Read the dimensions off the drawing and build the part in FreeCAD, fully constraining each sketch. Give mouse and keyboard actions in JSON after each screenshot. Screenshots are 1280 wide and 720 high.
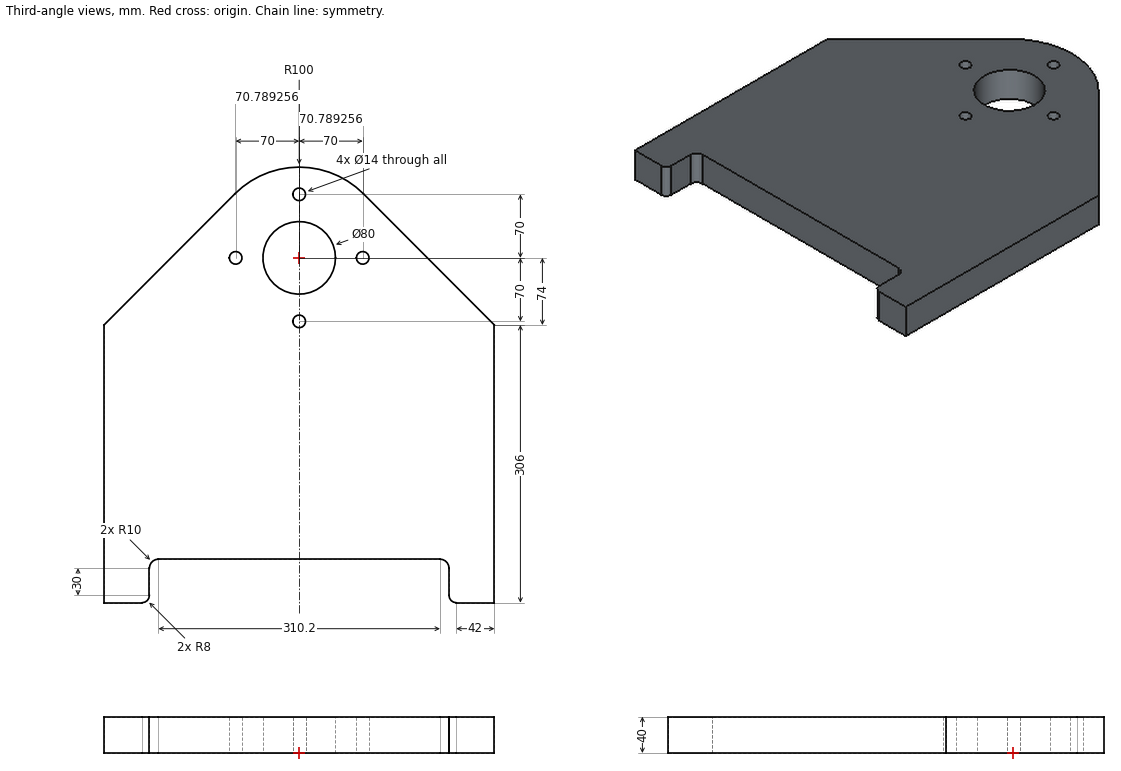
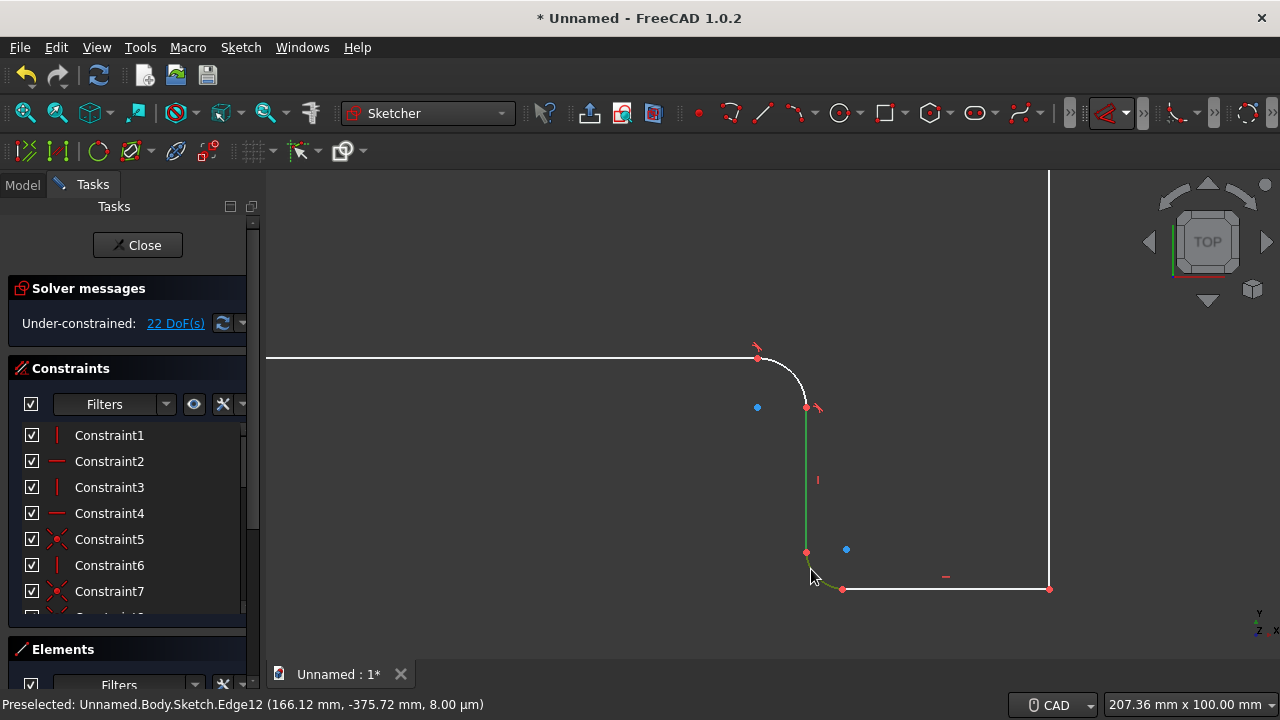
{"action": "key", "text": "t"}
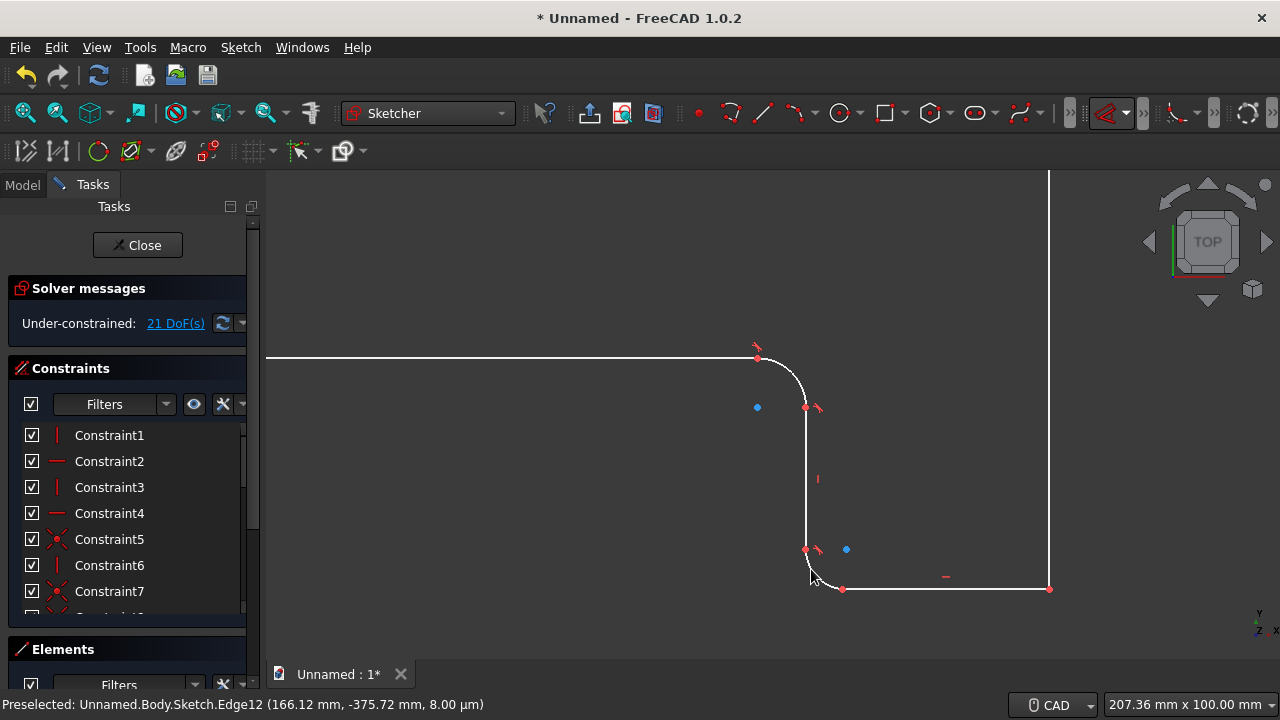
{"action": "scroll", "coordinate": [815, 571], "scroll_direction": "down", "scroll_amount": 10}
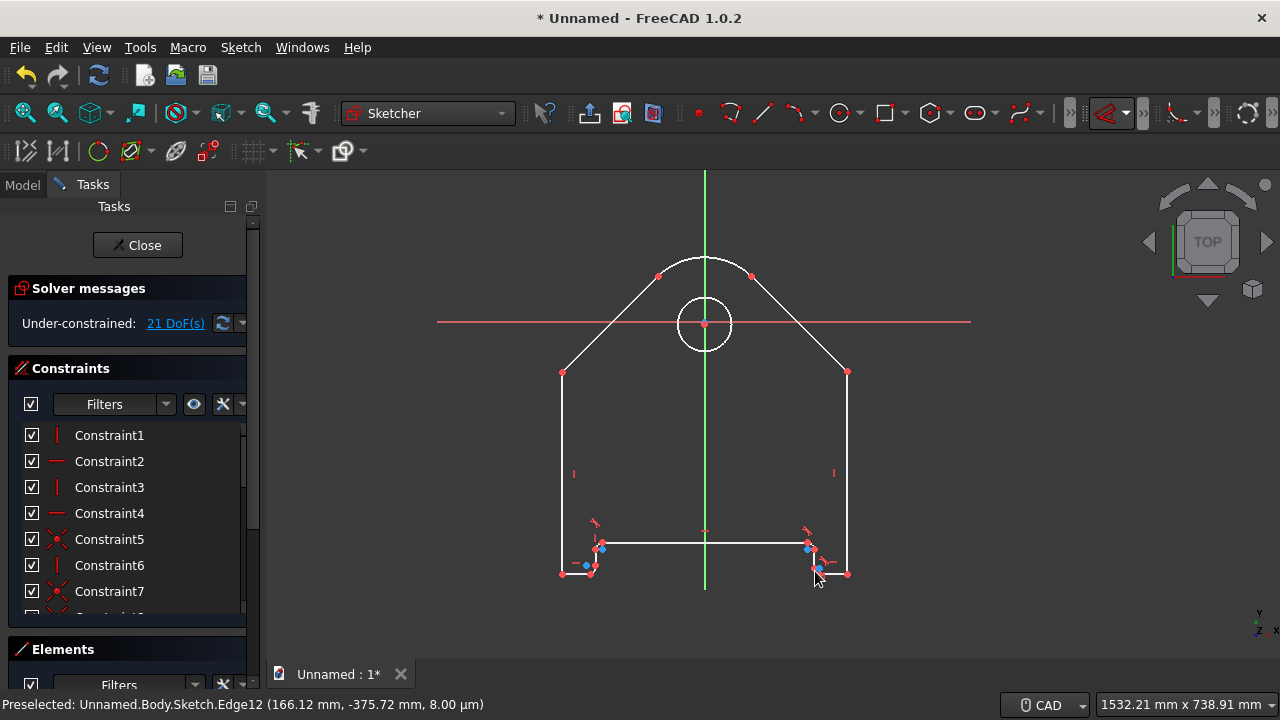
{"action": "scroll", "coordinate": [828, 574], "scroll_direction": "up", "scroll_amount": 3}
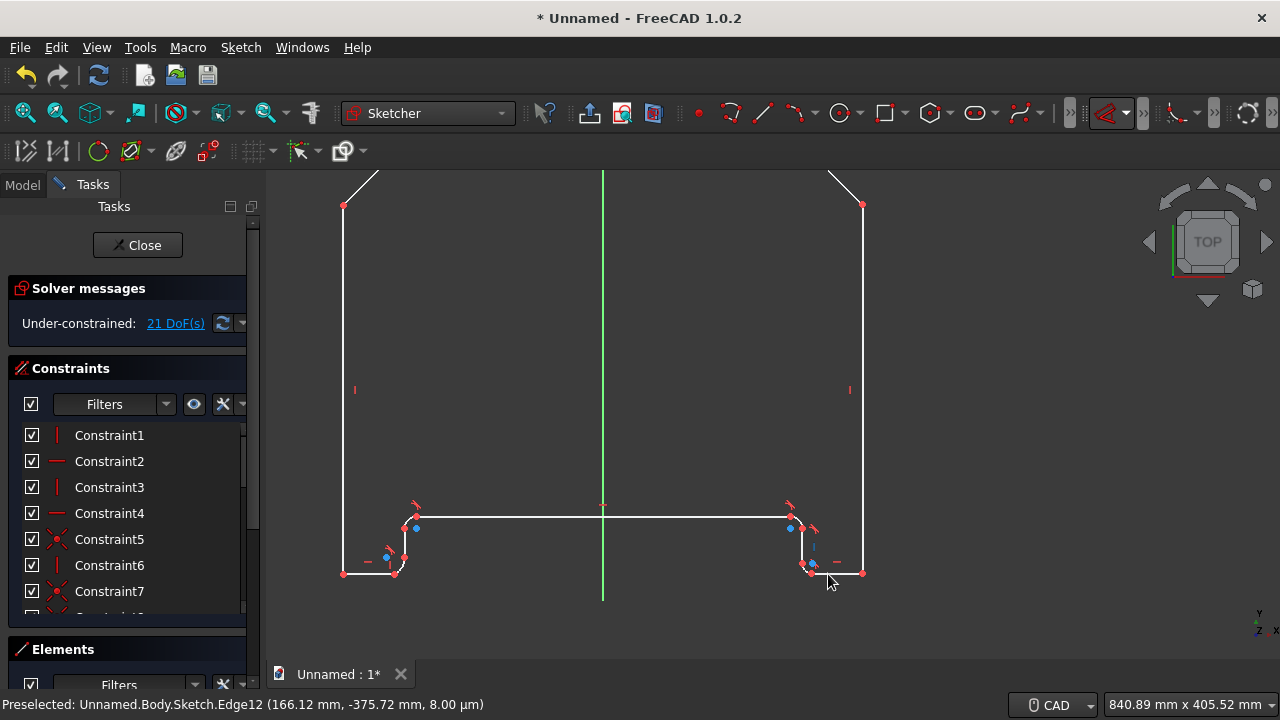
{"action": "left_click", "coordinate": [827, 574]}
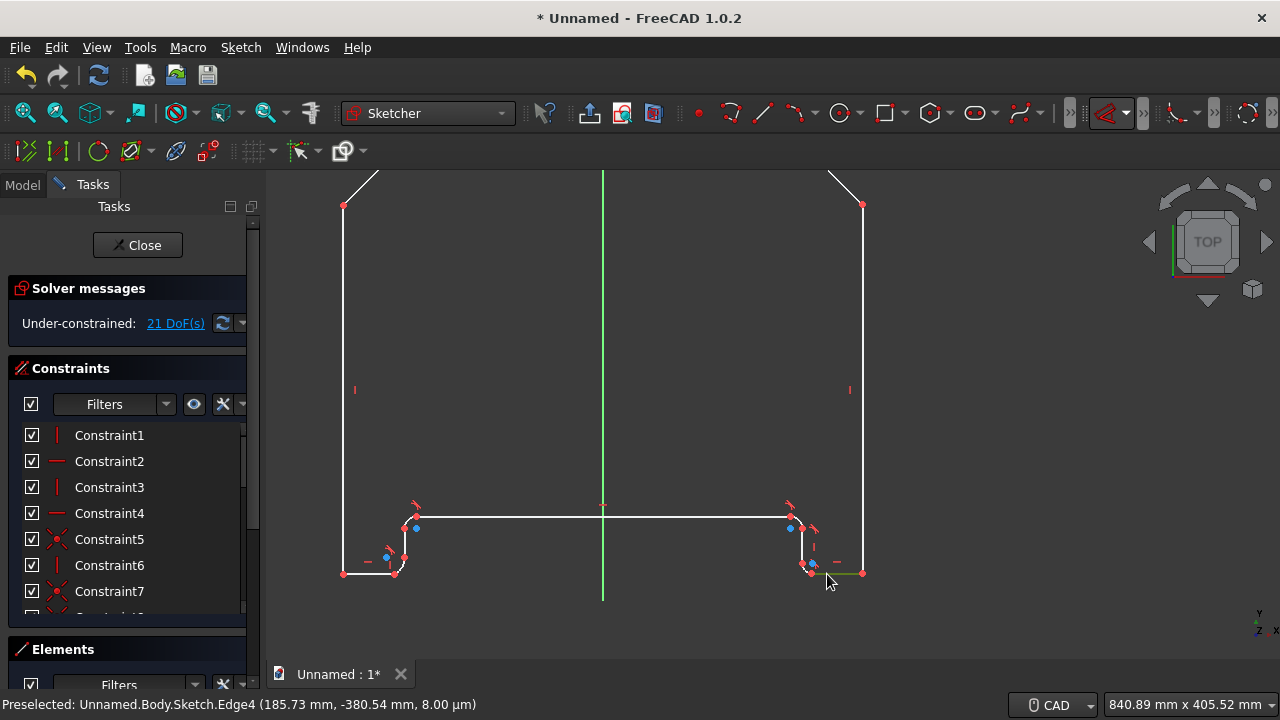
{"action": "scroll", "coordinate": [805, 570], "scroll_direction": "up", "scroll_amount": 4}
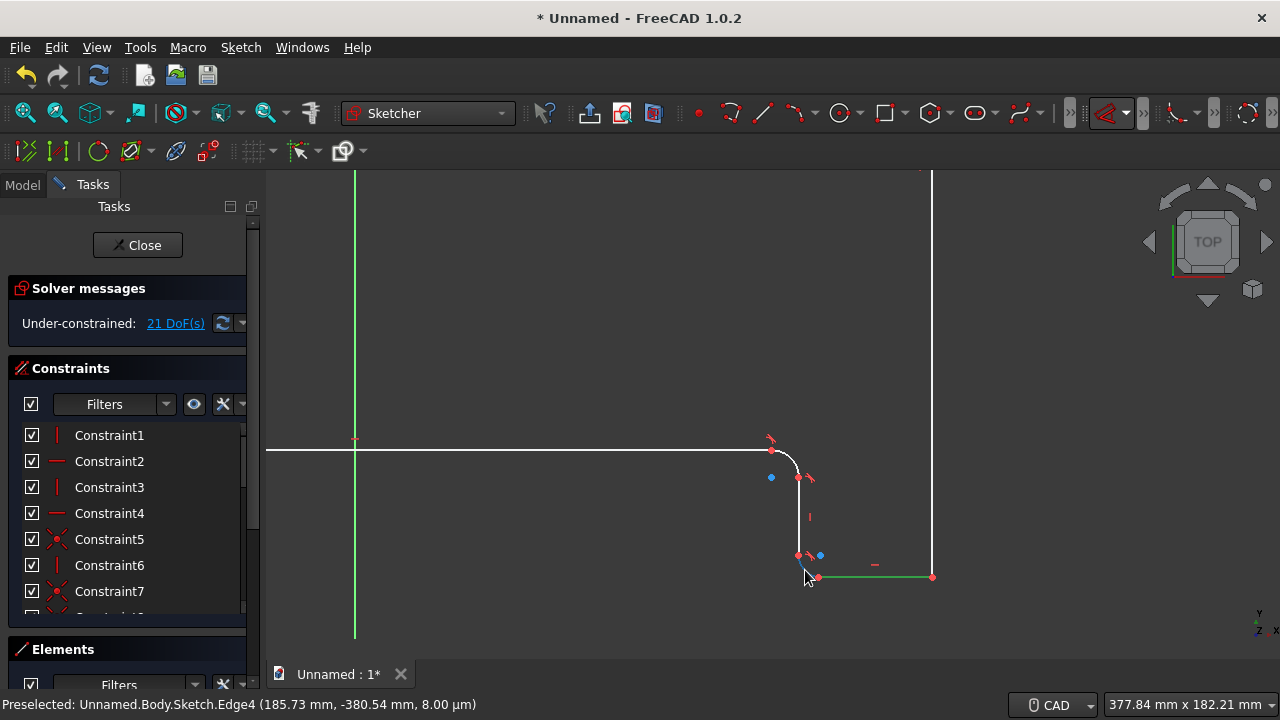
{"action": "left_click", "coordinate": [805, 570]}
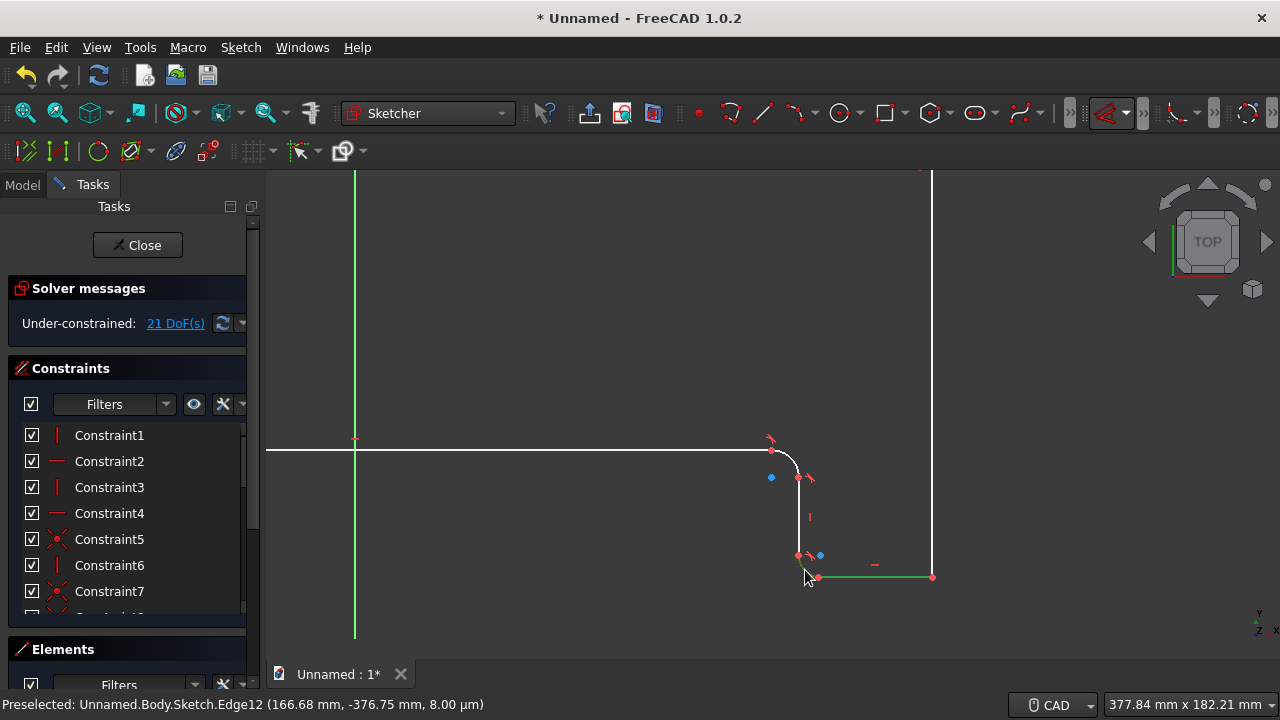
{"action": "key", "text": "t"}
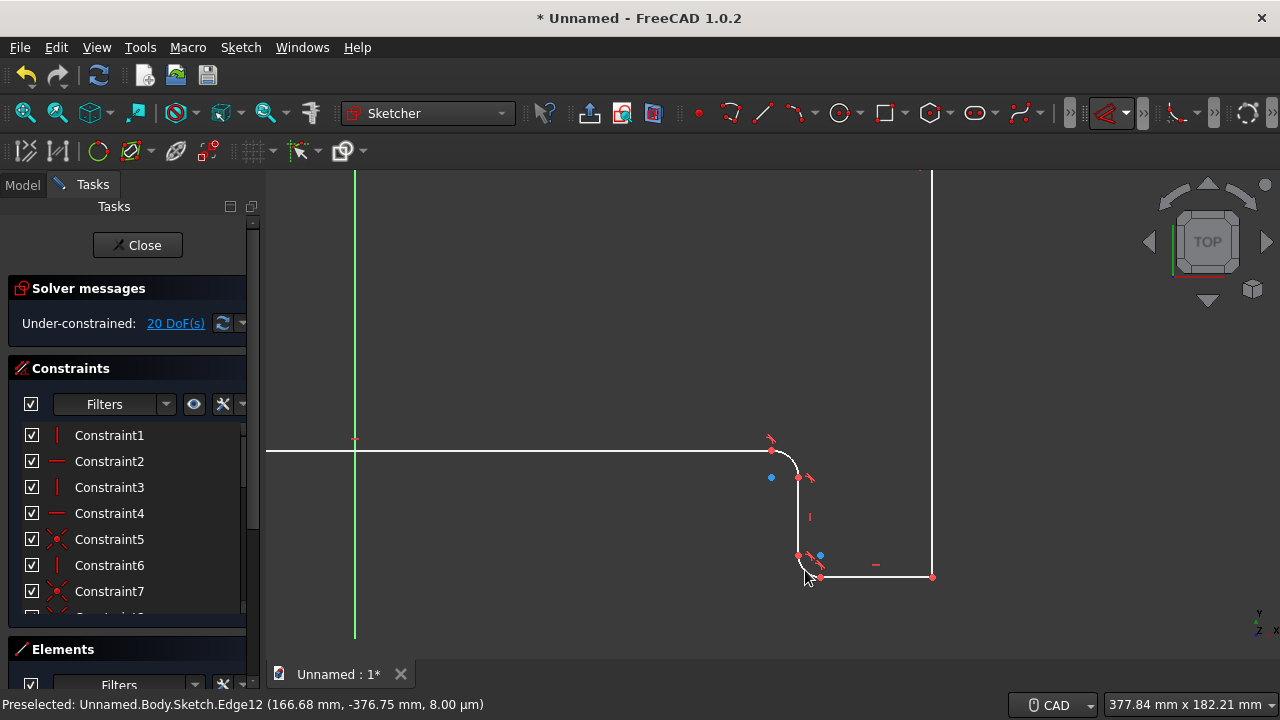
{"action": "scroll", "coordinate": [819, 573], "scroll_direction": "down", "scroll_amount": 7}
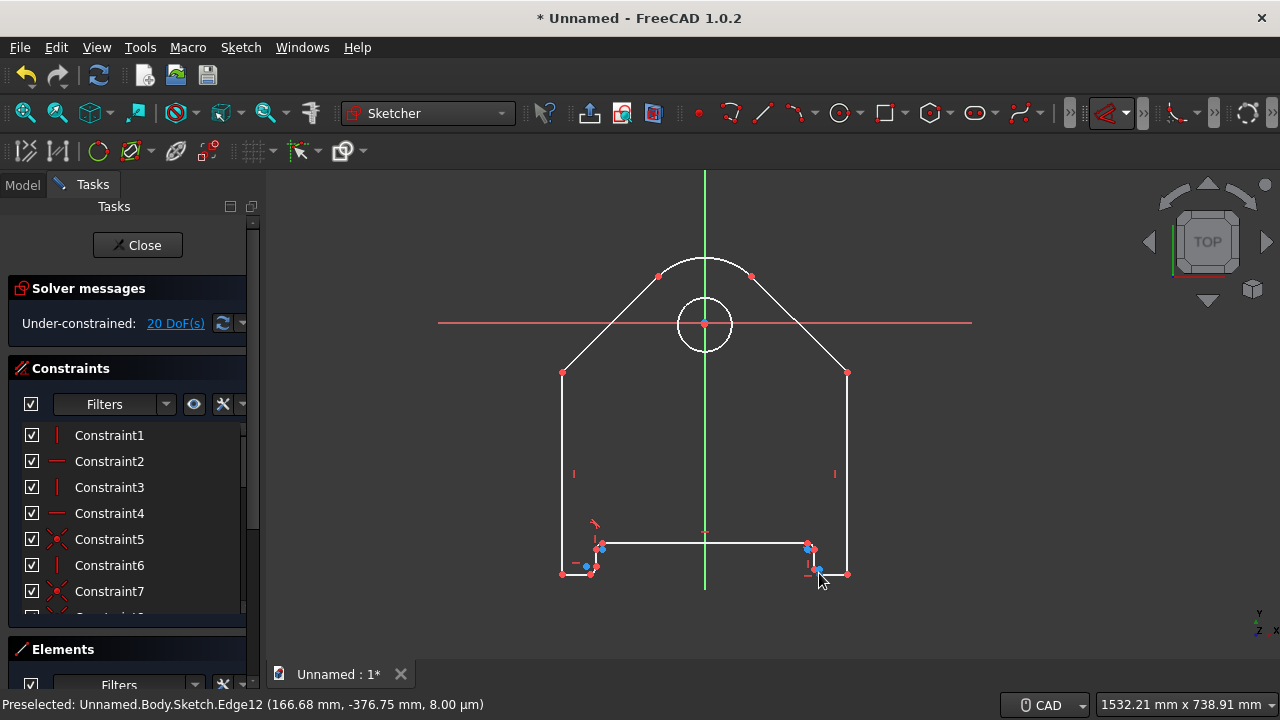
{"action": "scroll", "coordinate": [571, 575], "scroll_direction": "up", "scroll_amount": 3}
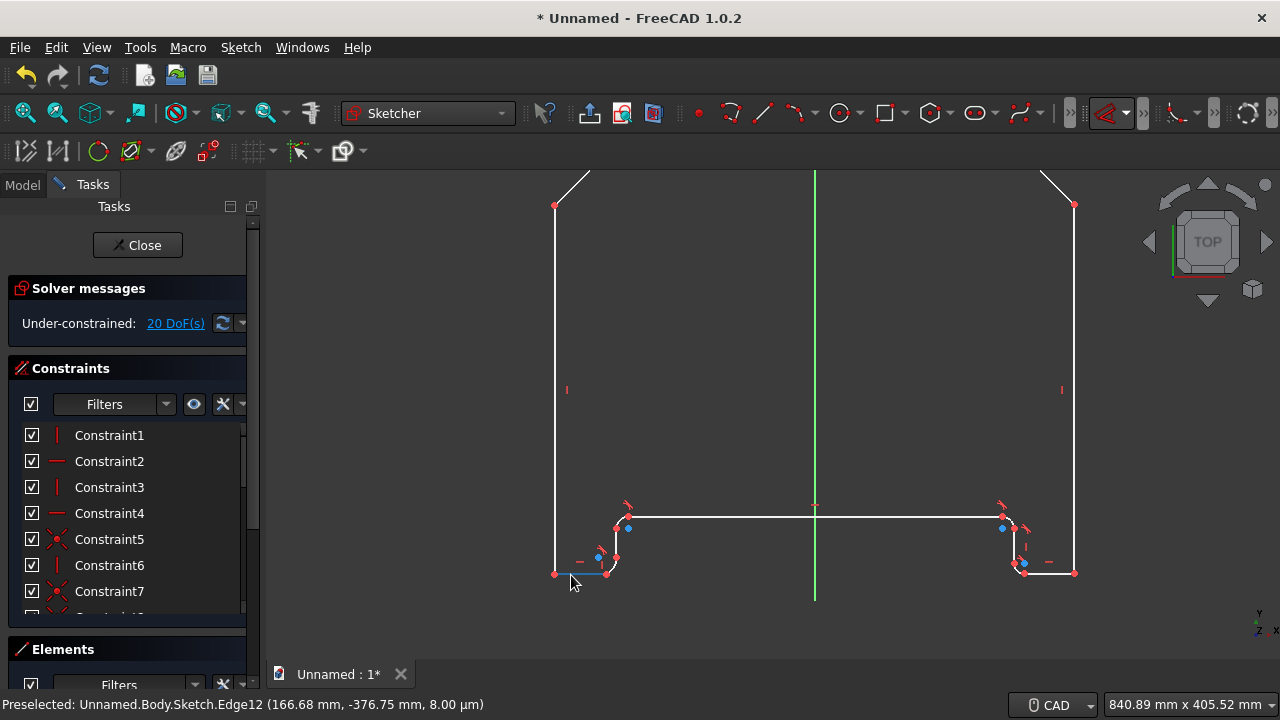
{"action": "left_click", "coordinate": [570, 574]}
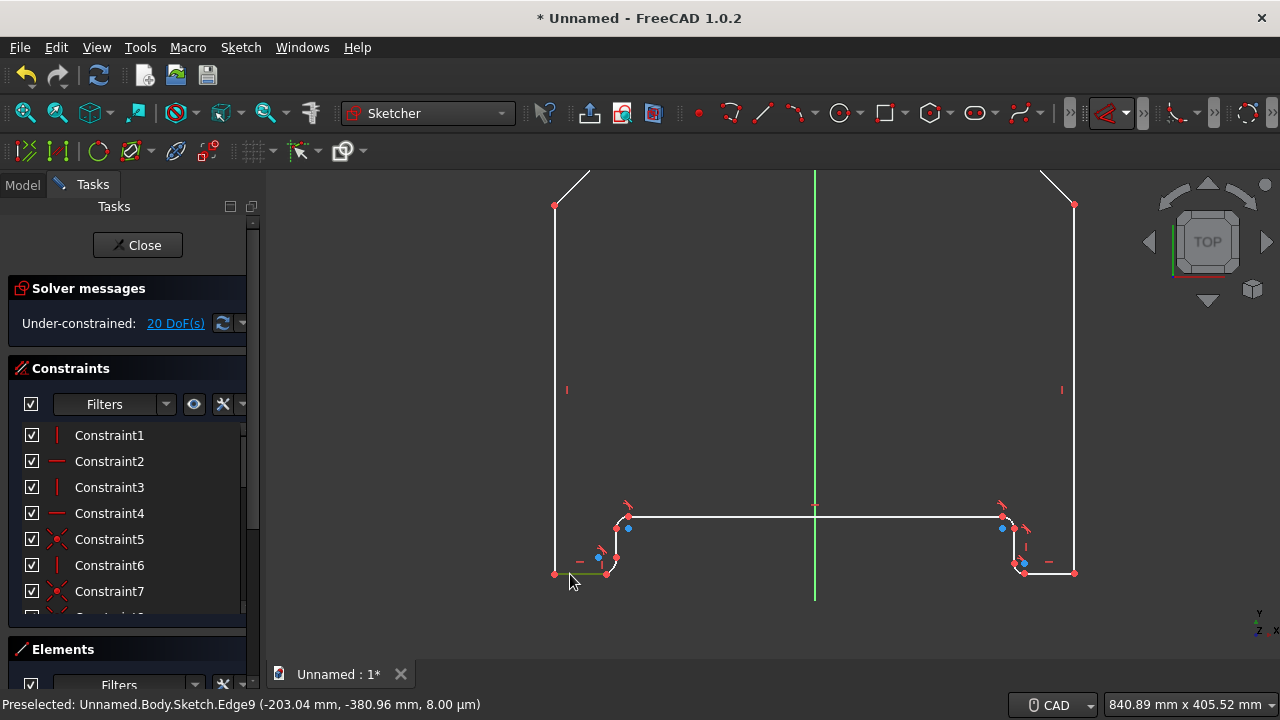
{"action": "scroll", "coordinate": [614, 568], "scroll_direction": "up", "scroll_amount": 2}